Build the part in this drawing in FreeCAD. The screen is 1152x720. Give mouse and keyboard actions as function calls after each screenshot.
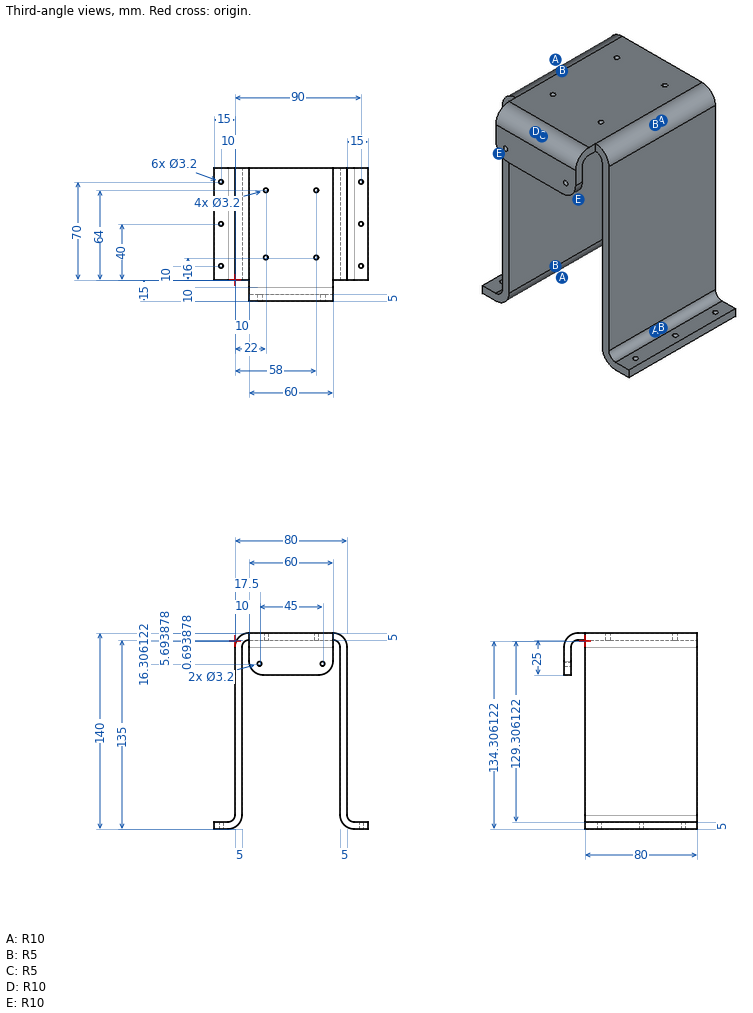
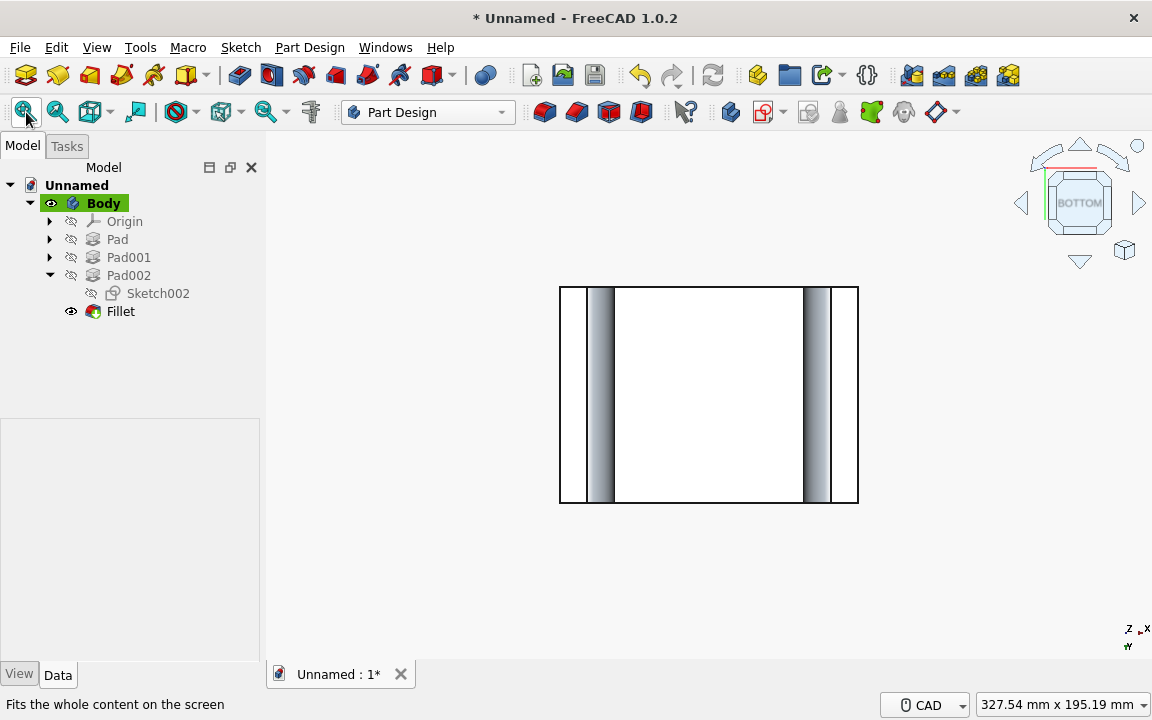
key(0)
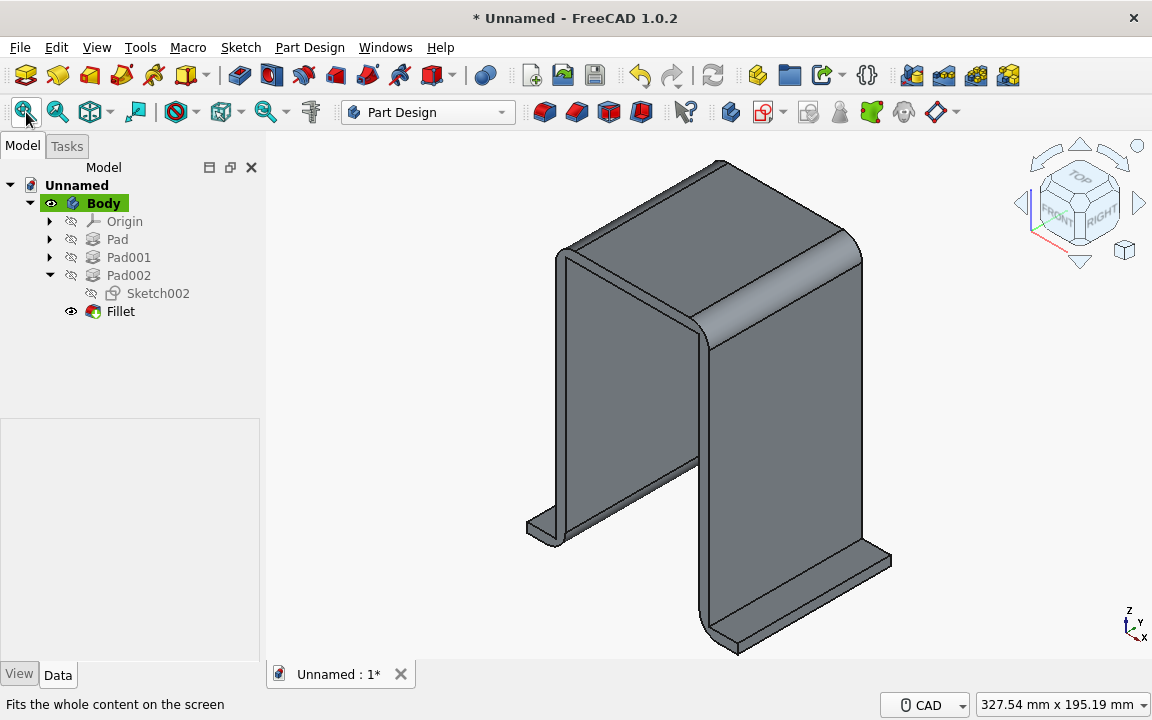
key(2)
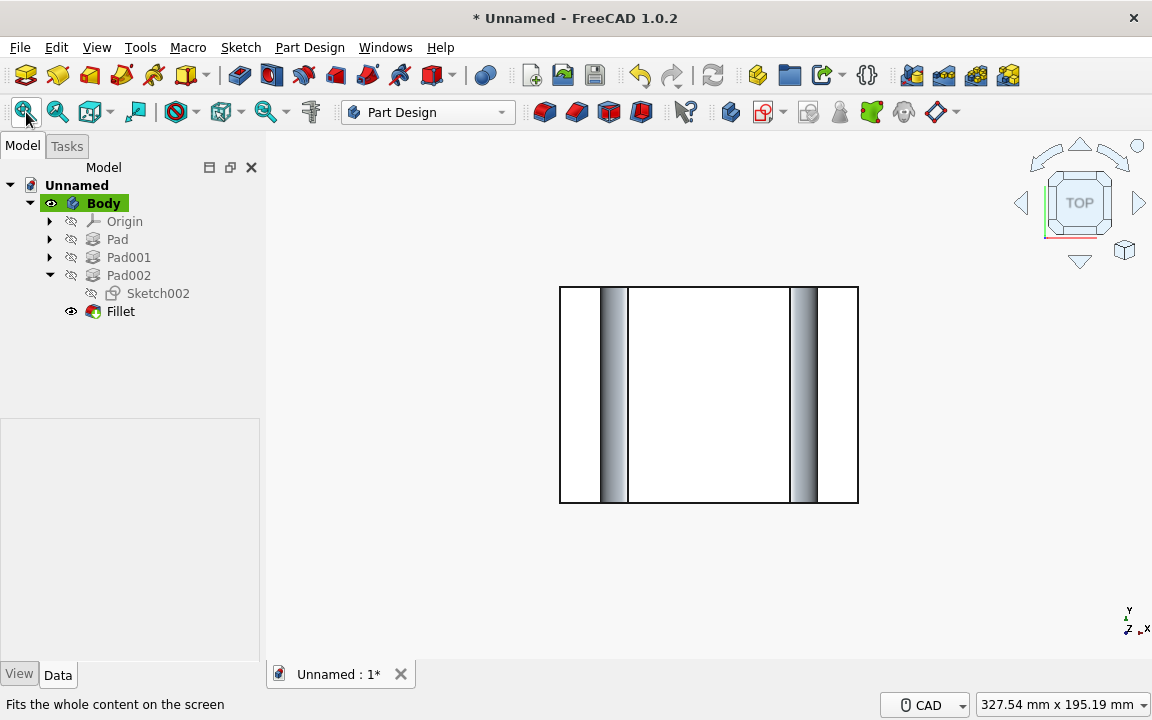
click(26, 112)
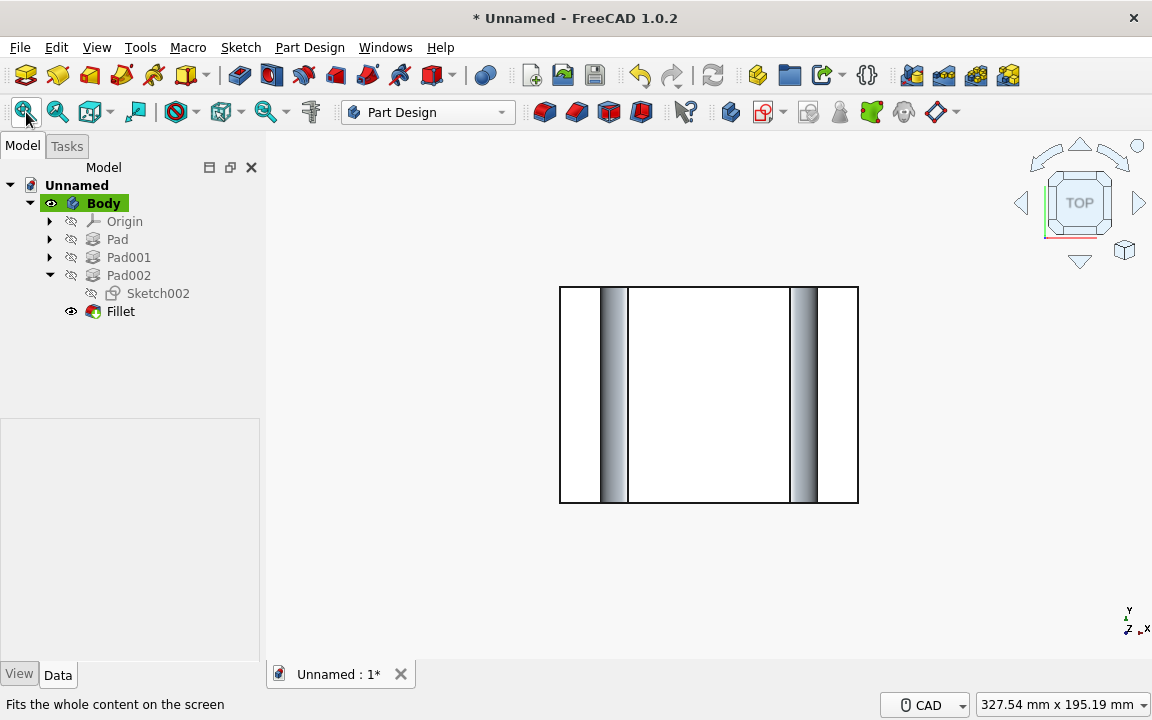
key(1)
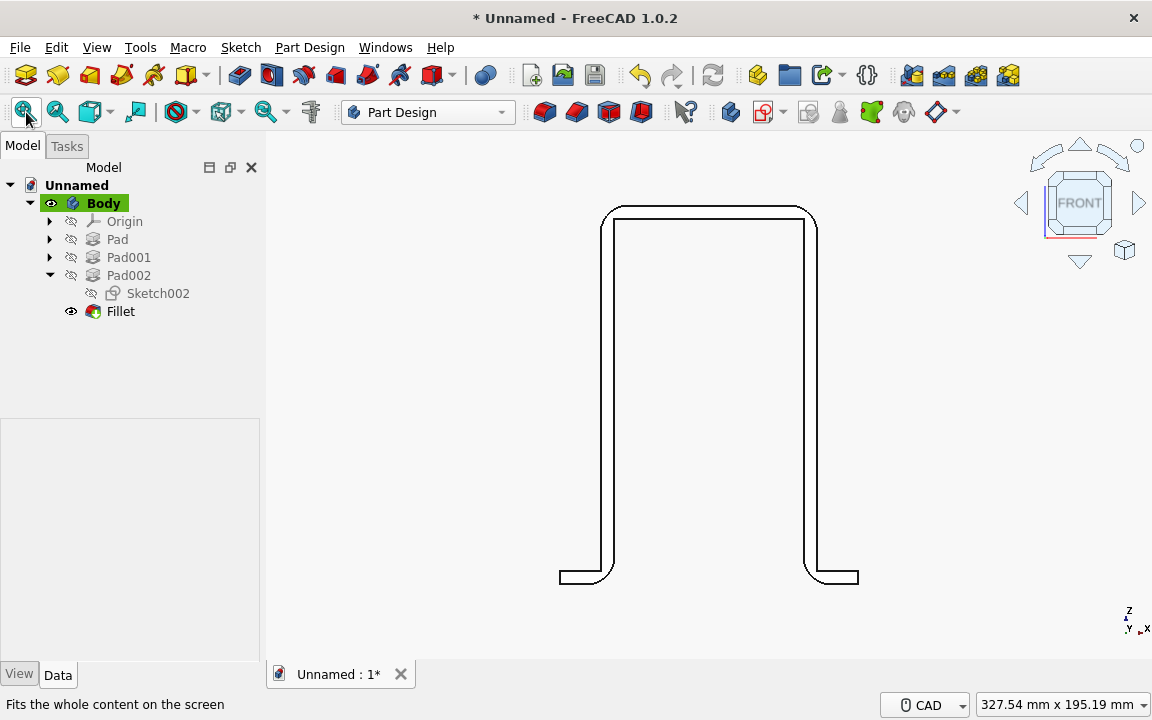
key(3)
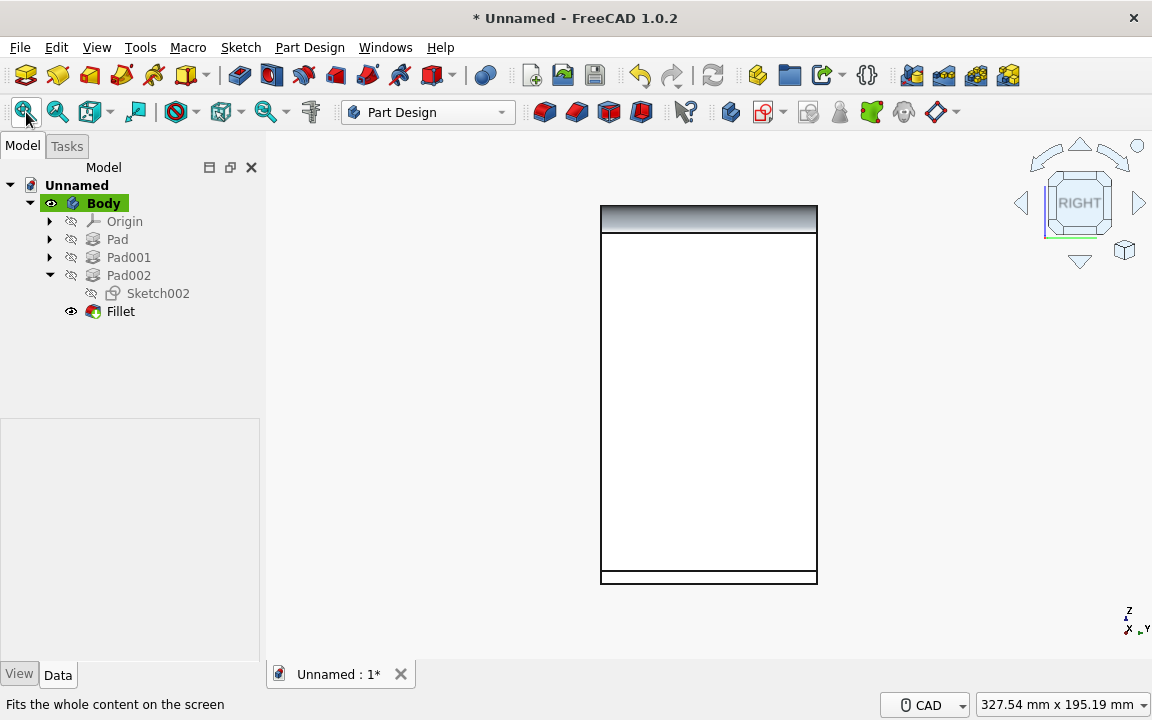
key(5)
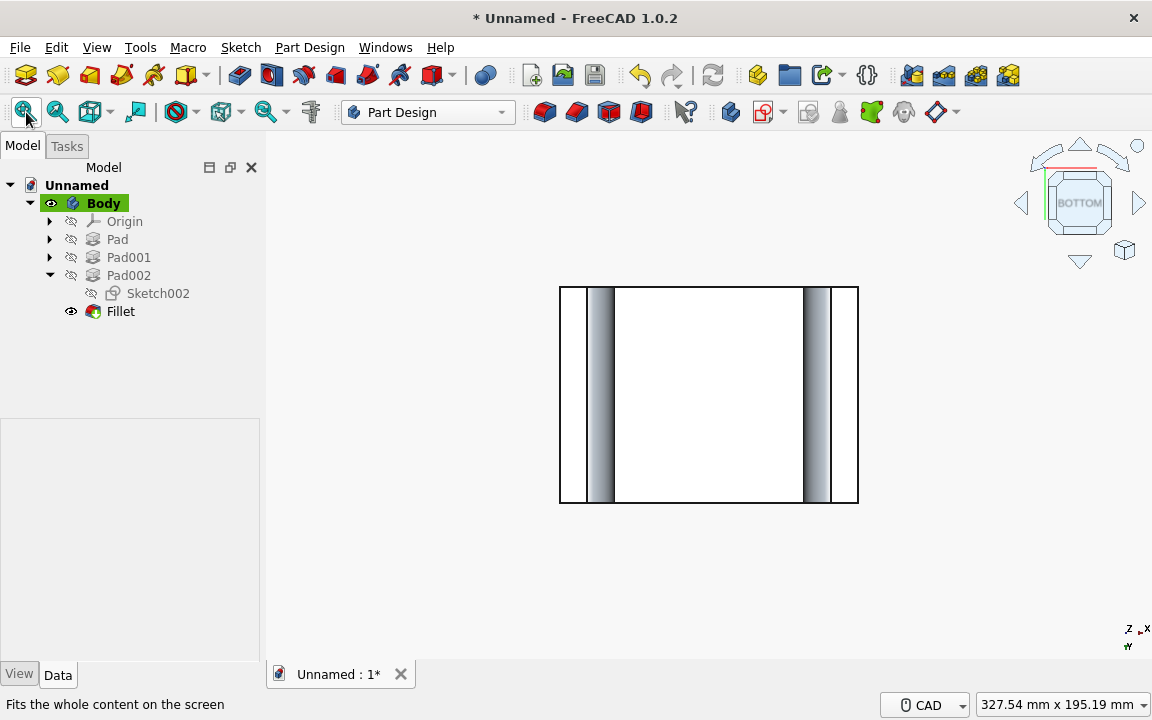
click(26, 112)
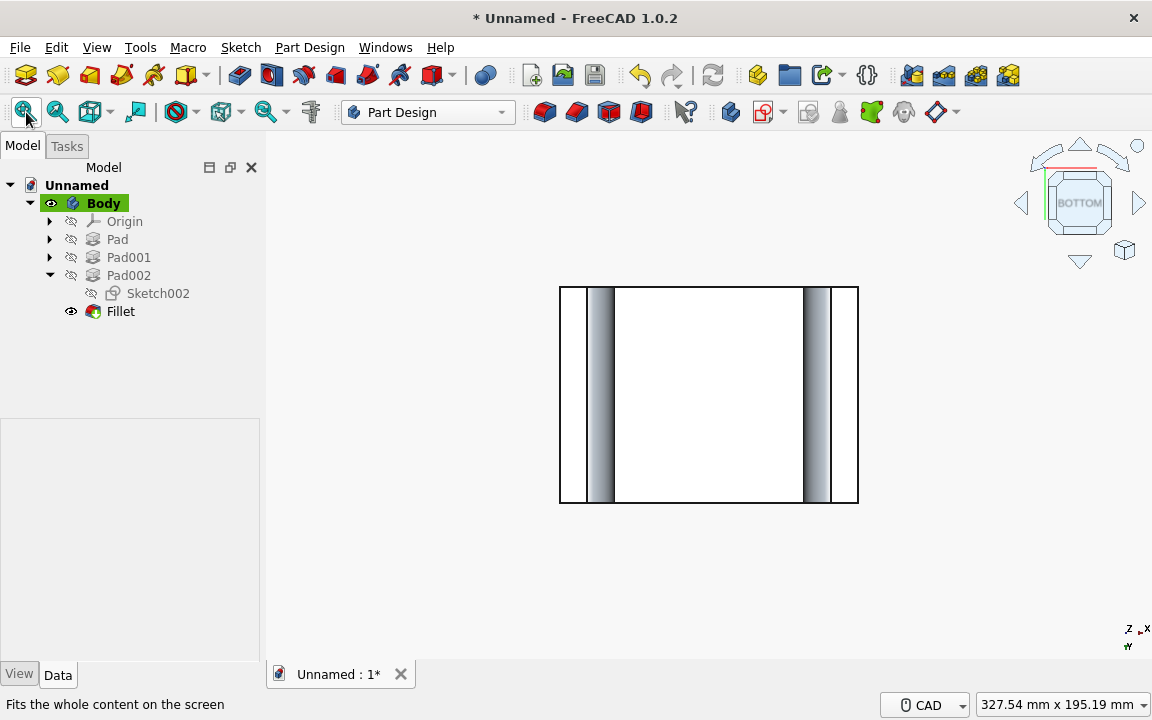
key(4)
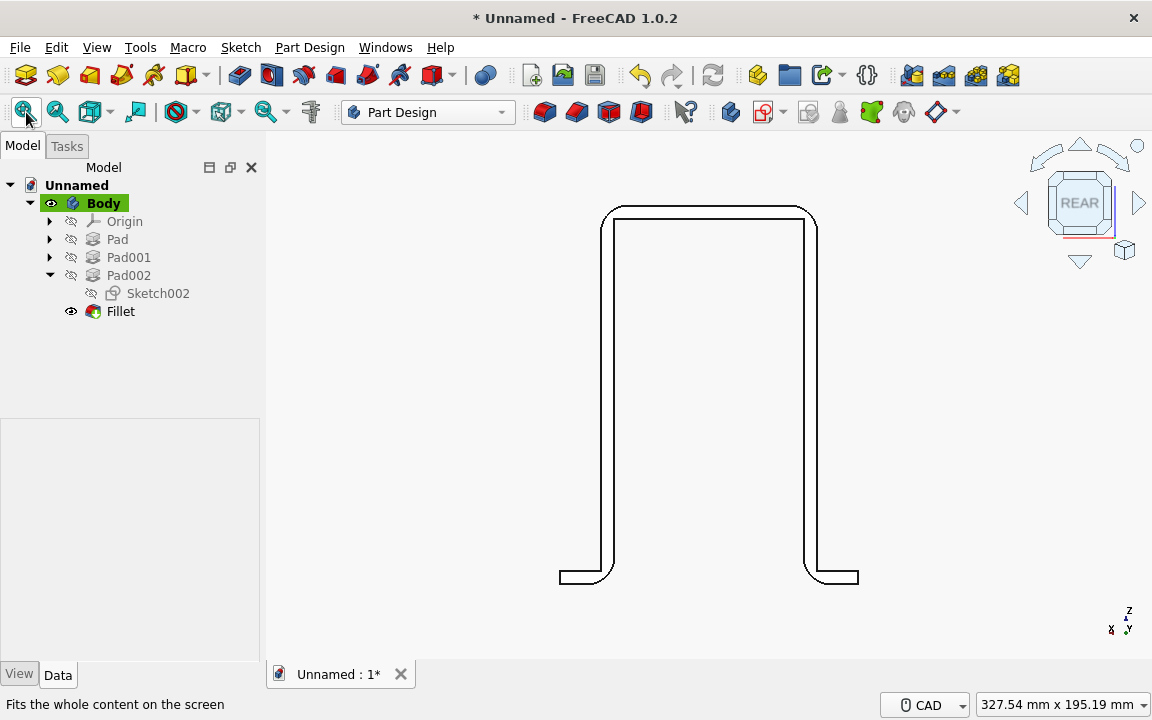
key(6)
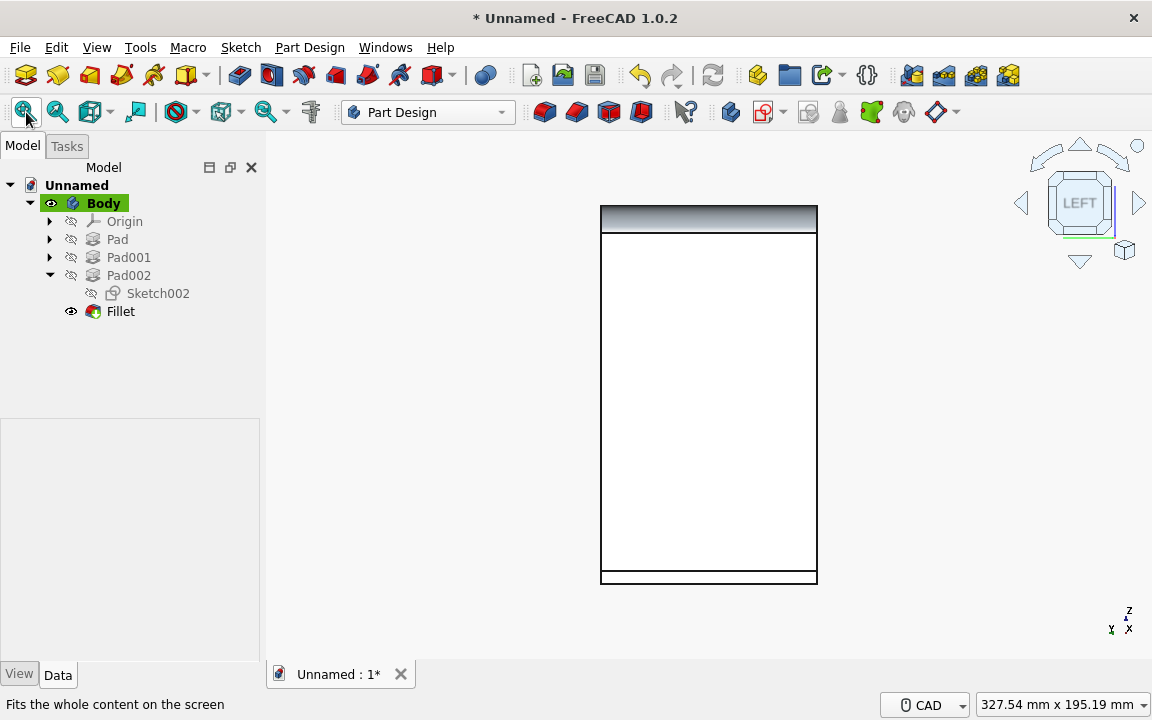
key(v)
key(3)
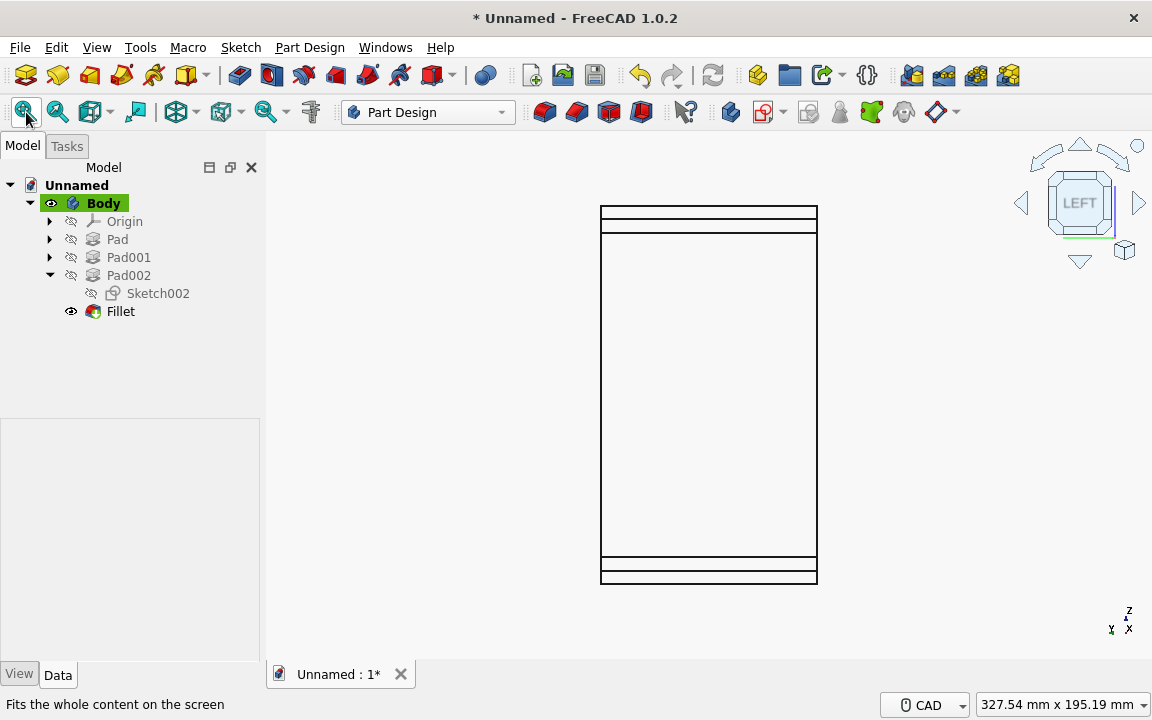
key(0)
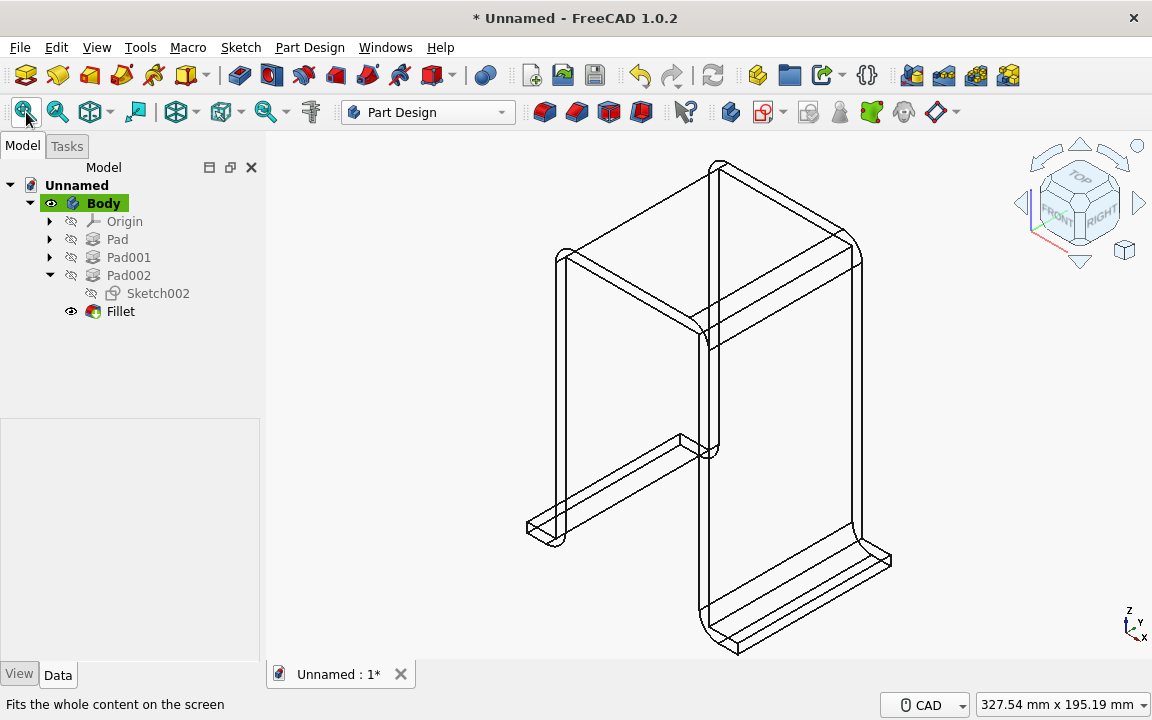
click(776, 289)